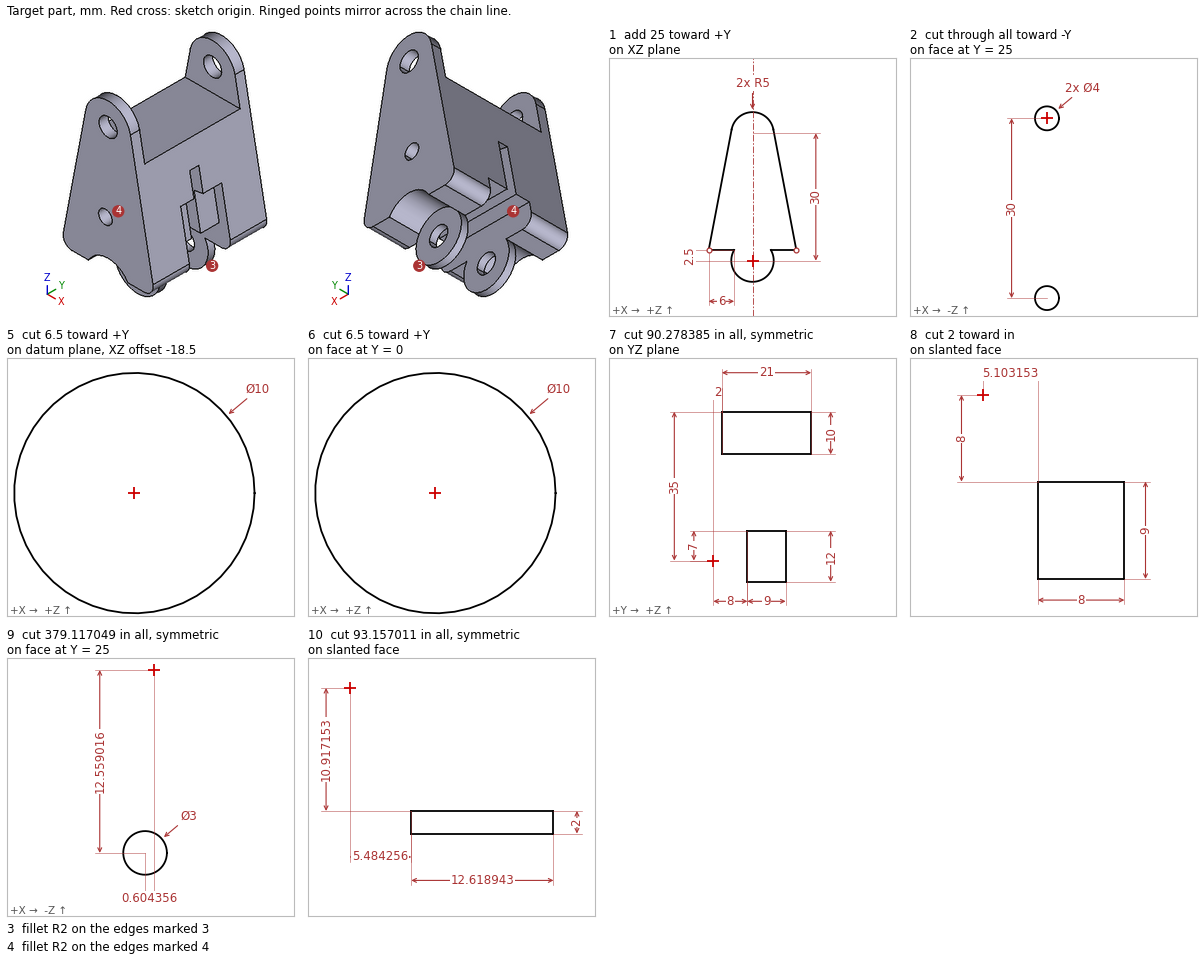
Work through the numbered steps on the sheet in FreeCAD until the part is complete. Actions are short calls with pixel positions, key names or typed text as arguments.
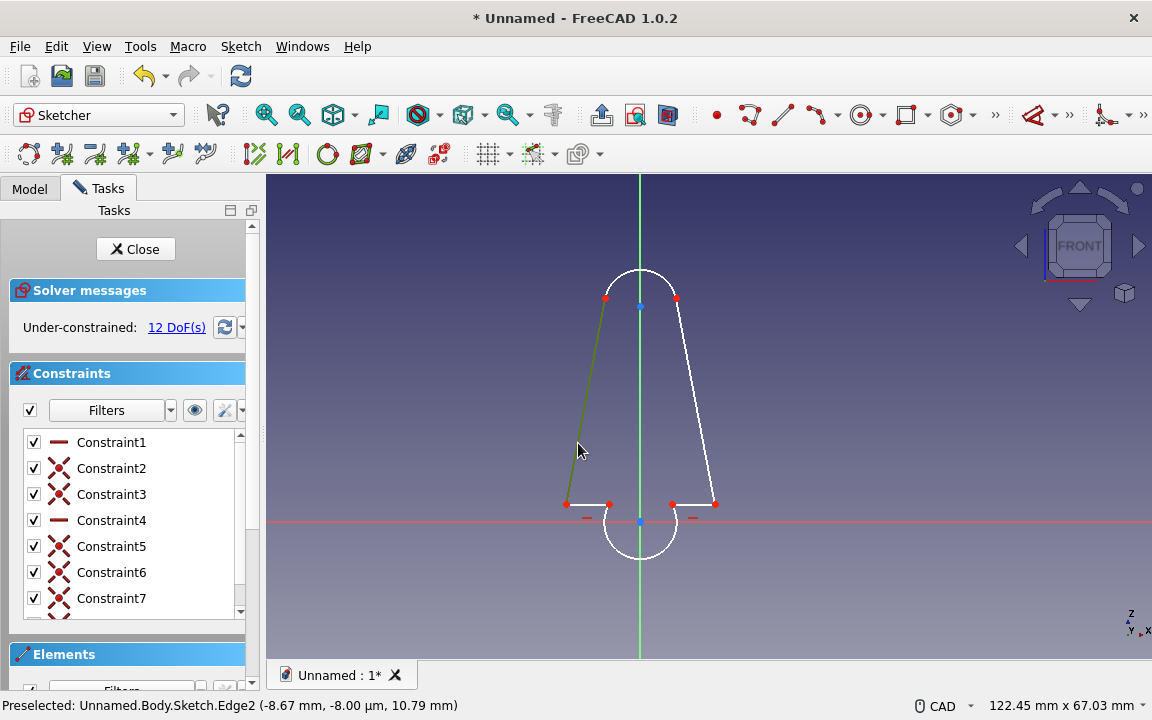
click(659, 275)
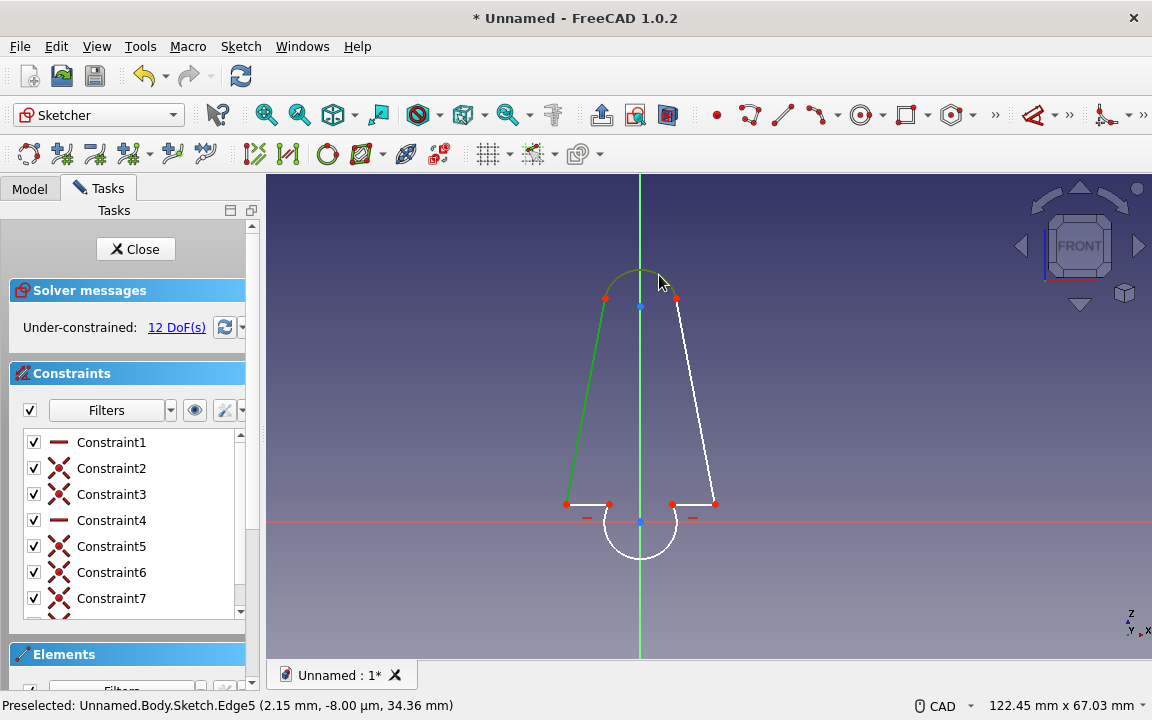
key(t)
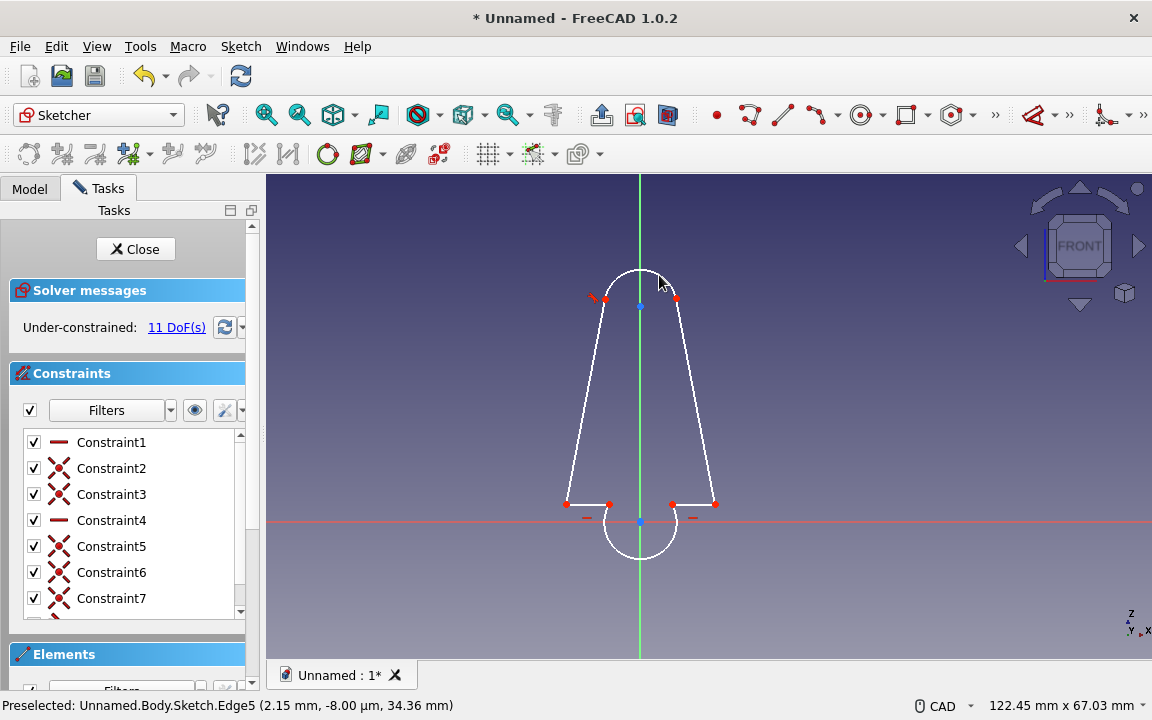
click(688, 361)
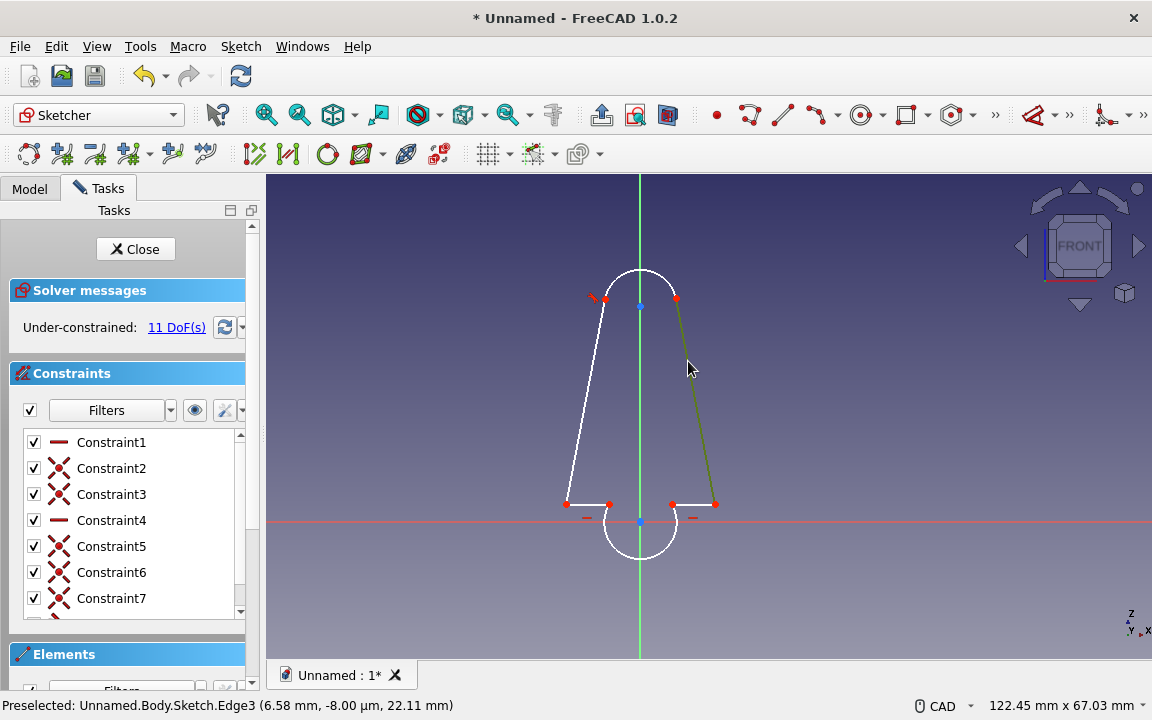
click(659, 275)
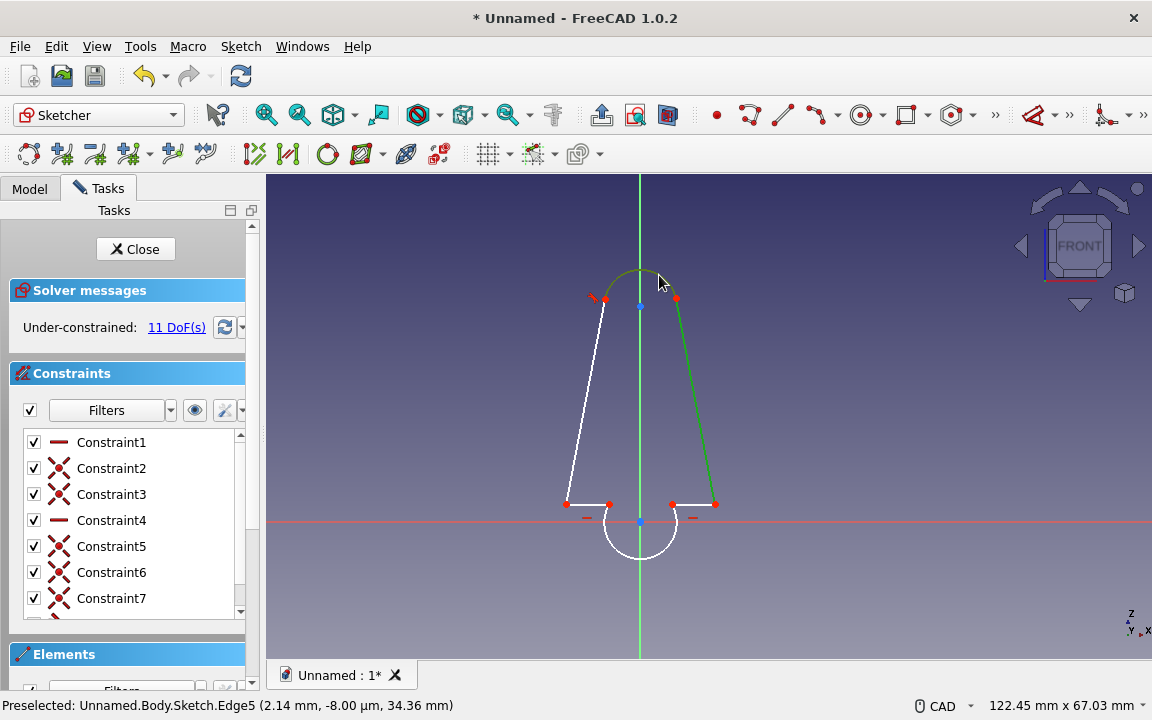
key(t)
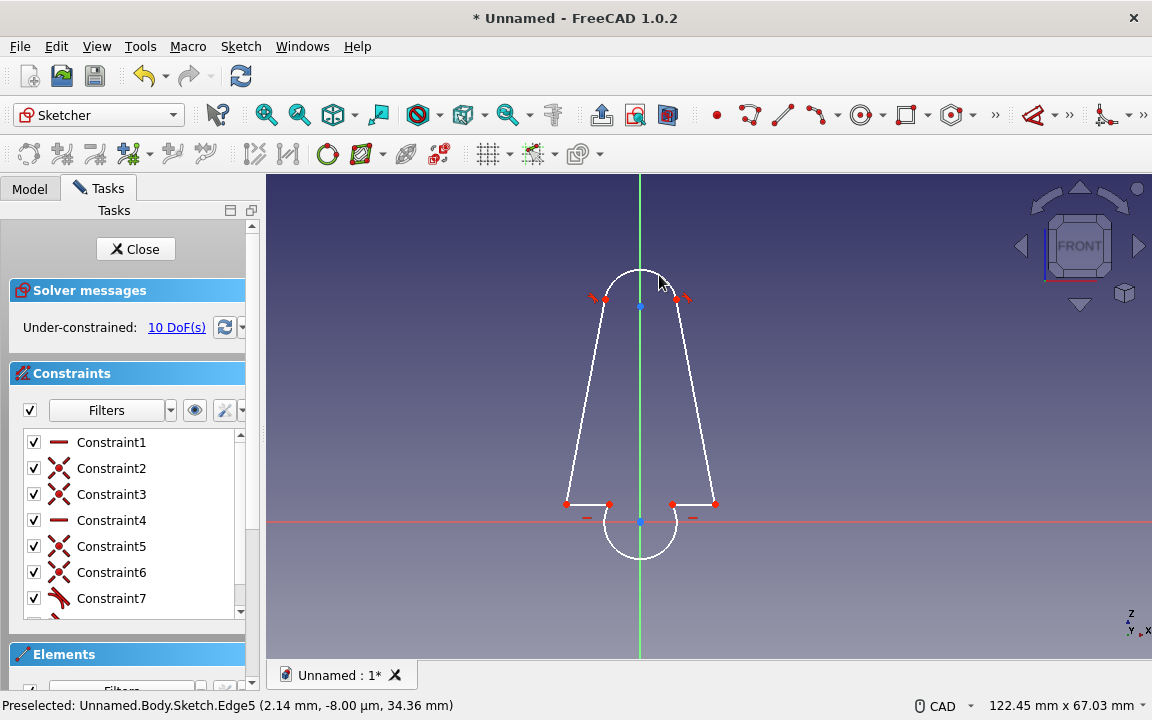
drag(630, 512, 651, 533)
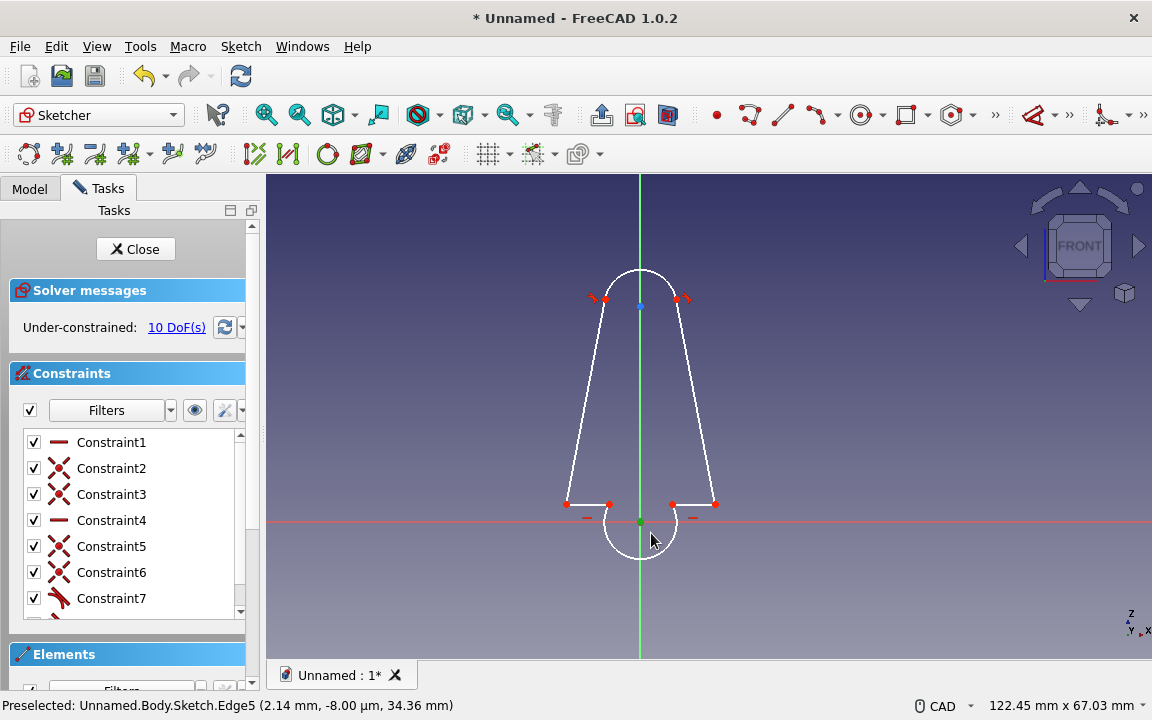
key(c)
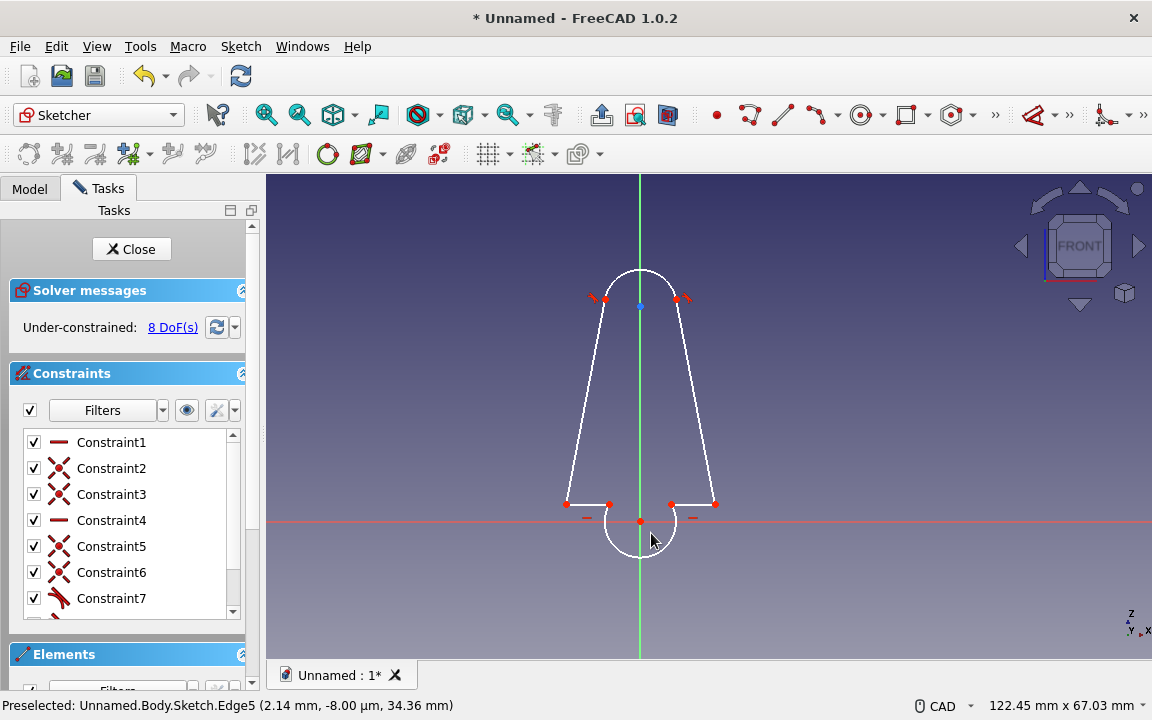
click(659, 275)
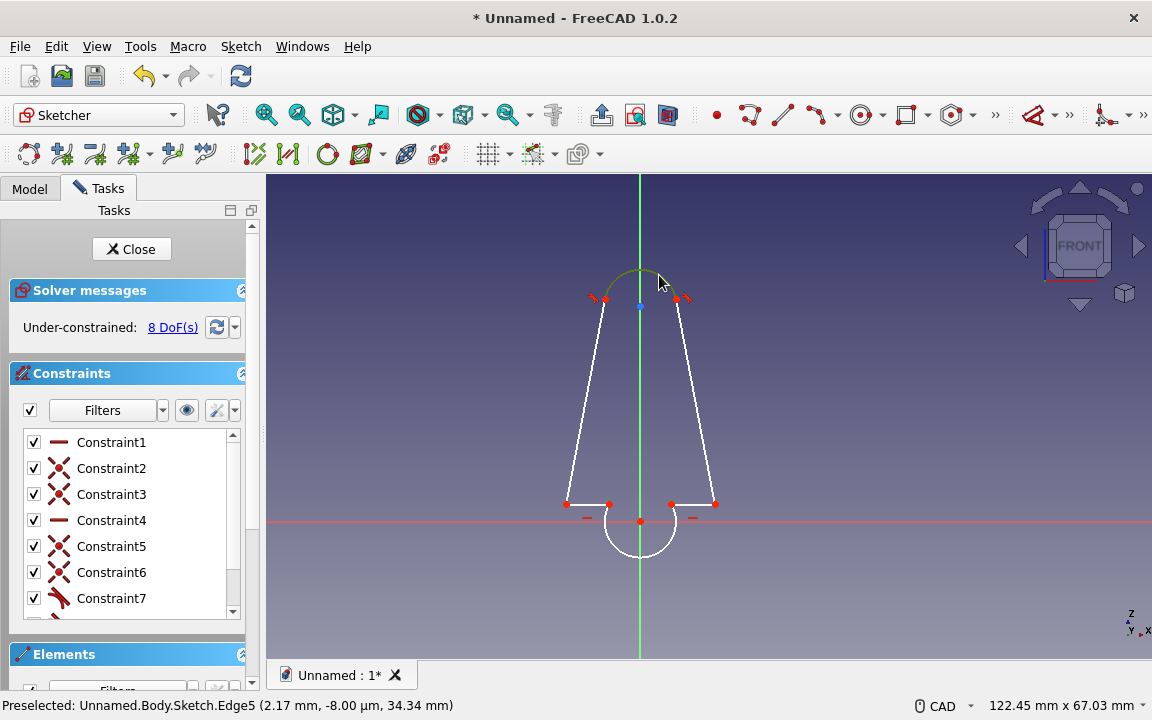
click(614, 546)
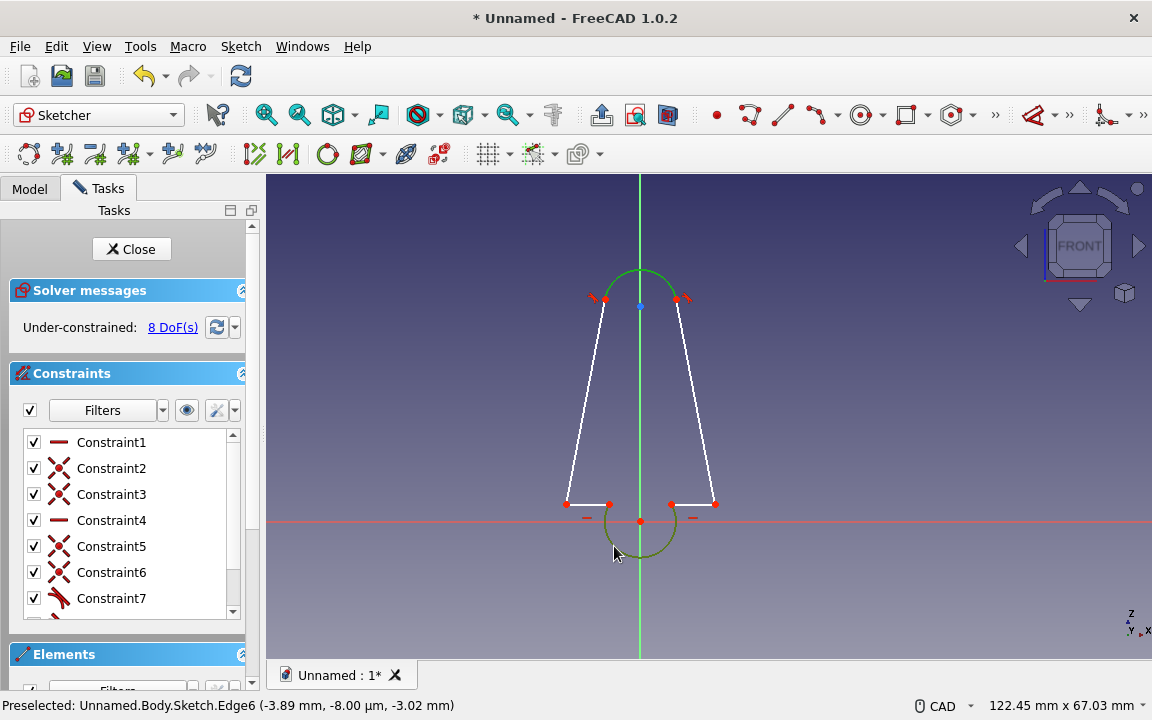
key(e)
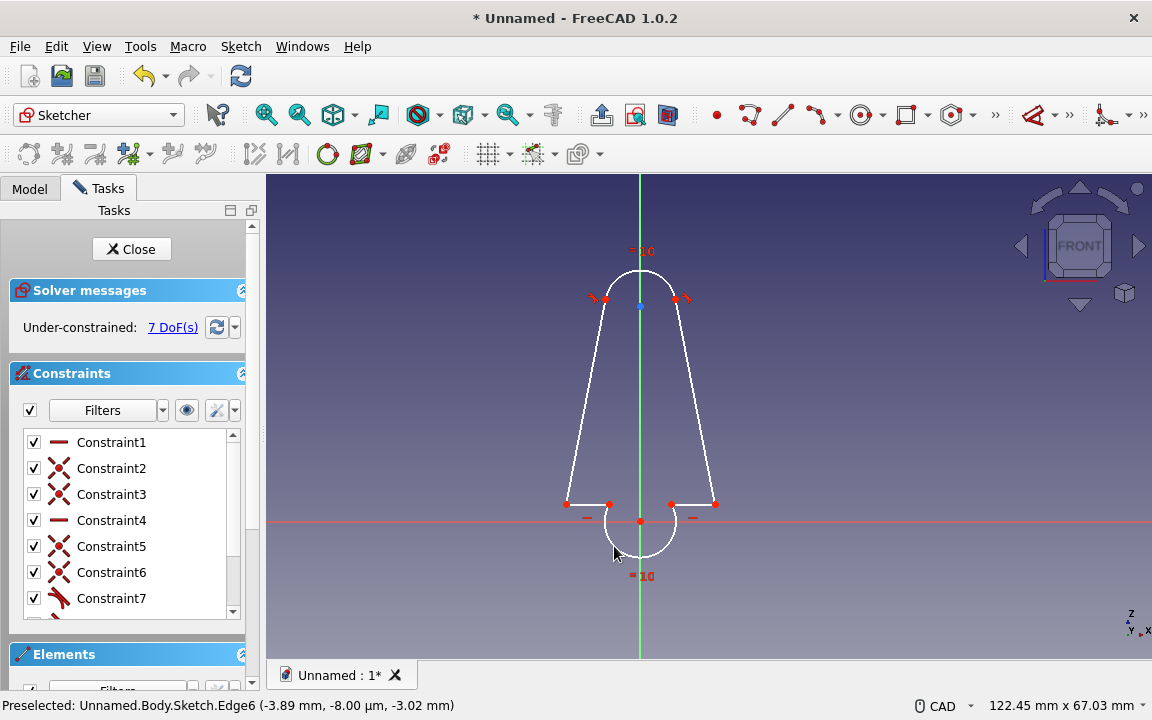
click(641, 306)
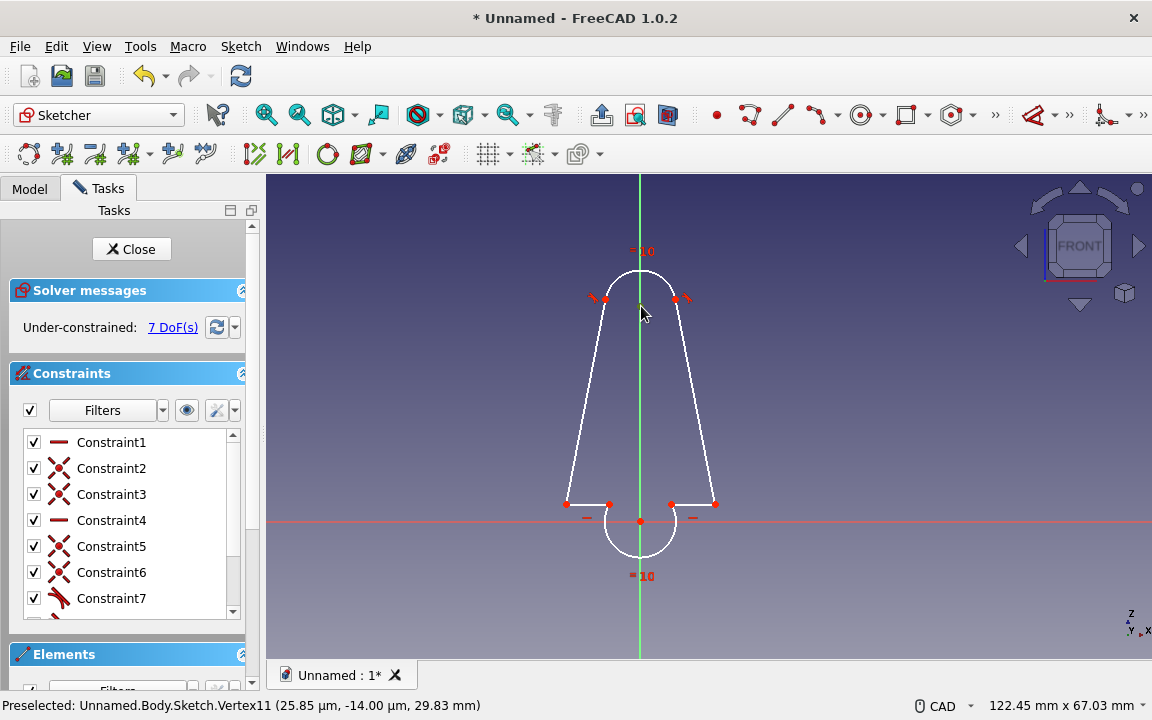
click(640, 600)